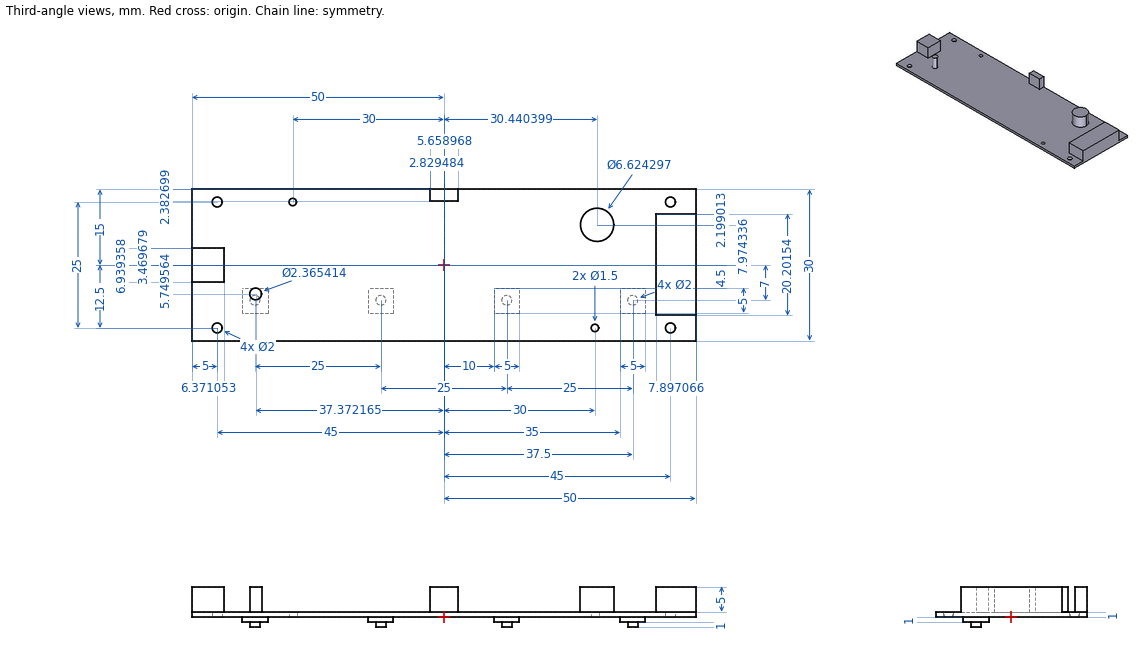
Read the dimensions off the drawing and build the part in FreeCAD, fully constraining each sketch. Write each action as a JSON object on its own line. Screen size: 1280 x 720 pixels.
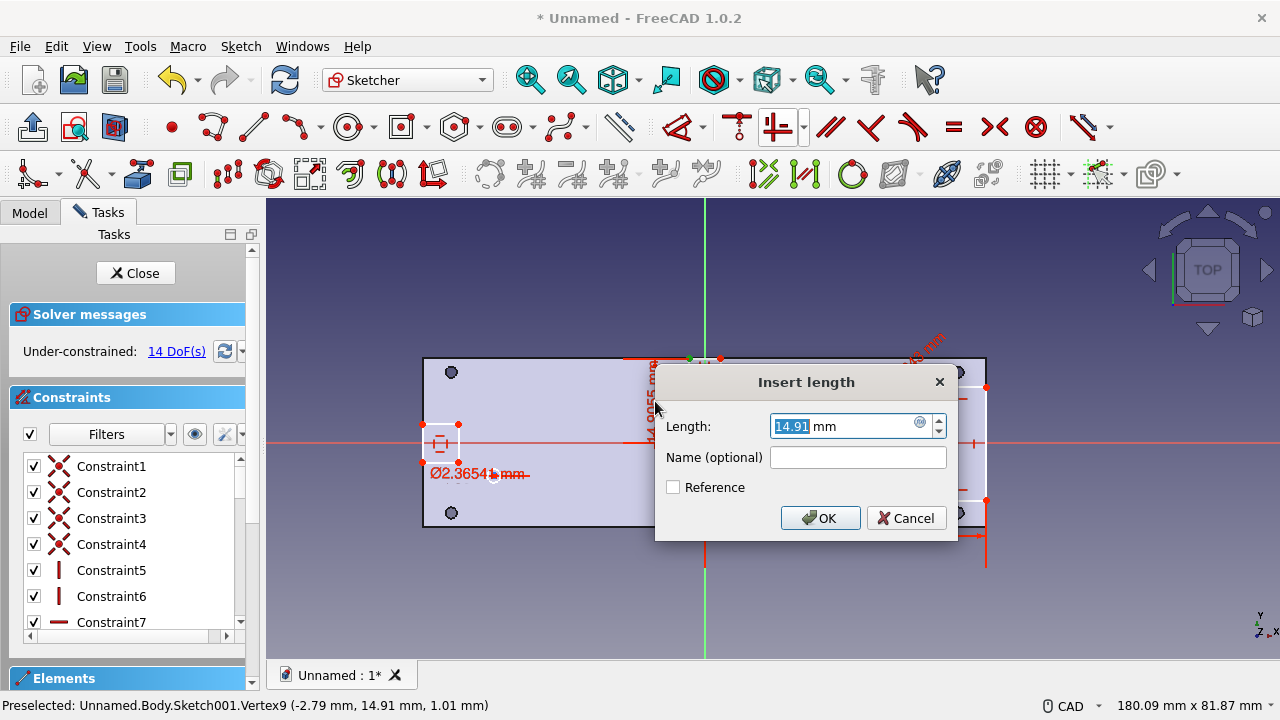
{"action": "type", "text": "15"}
{"action": "key", "text": "Return"}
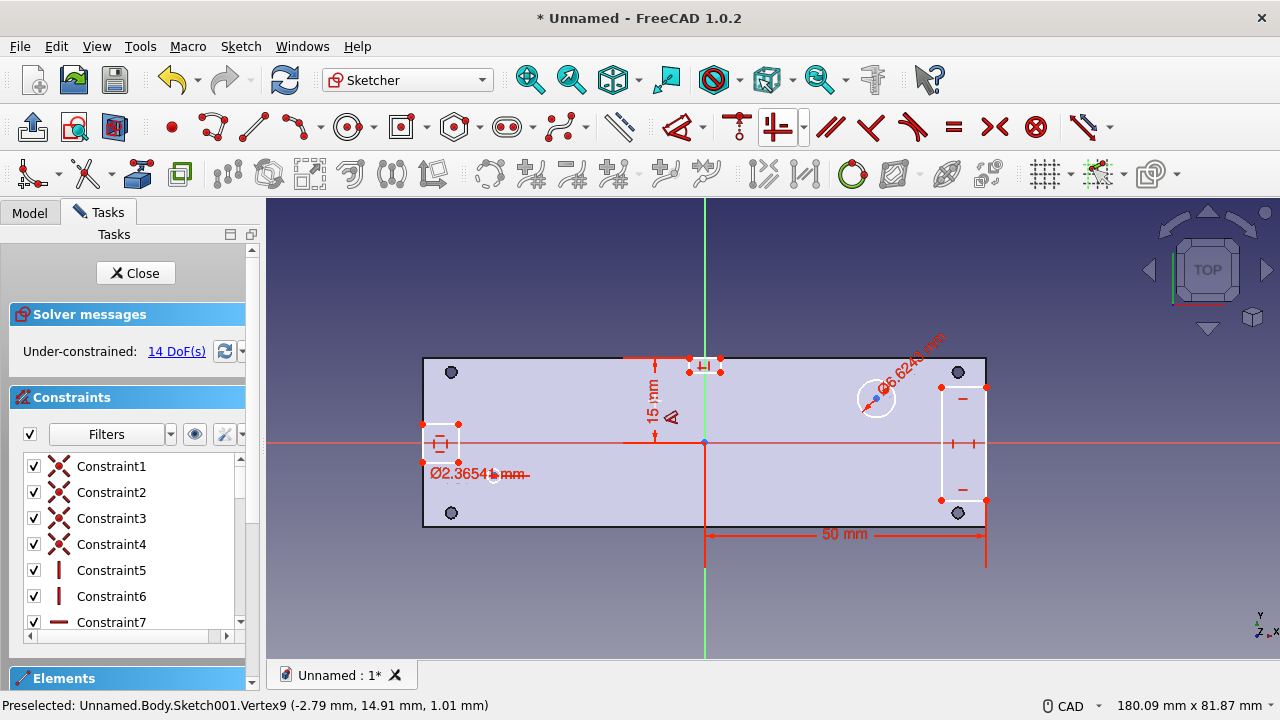
{"action": "left_click", "coordinate": [423, 424]}
{"action": "left_click", "coordinate": [564, 477]}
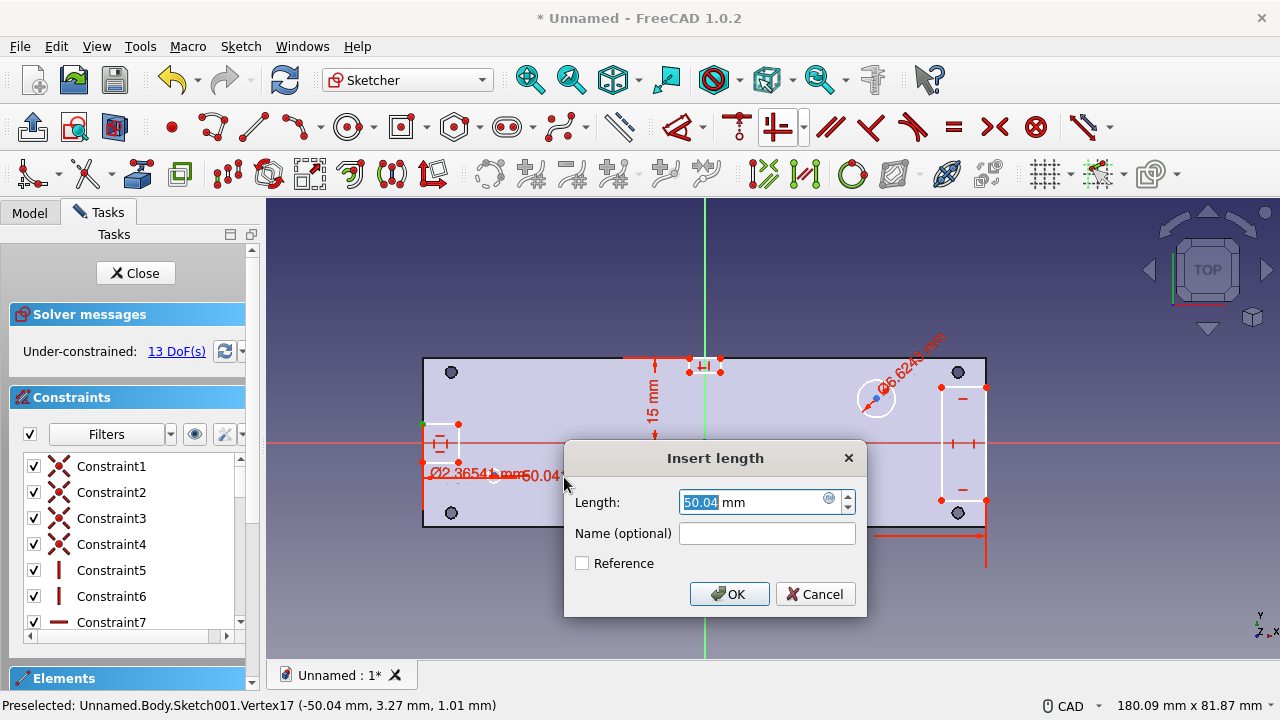
{"action": "type", "text": "50"}
{"action": "key", "text": "Return"}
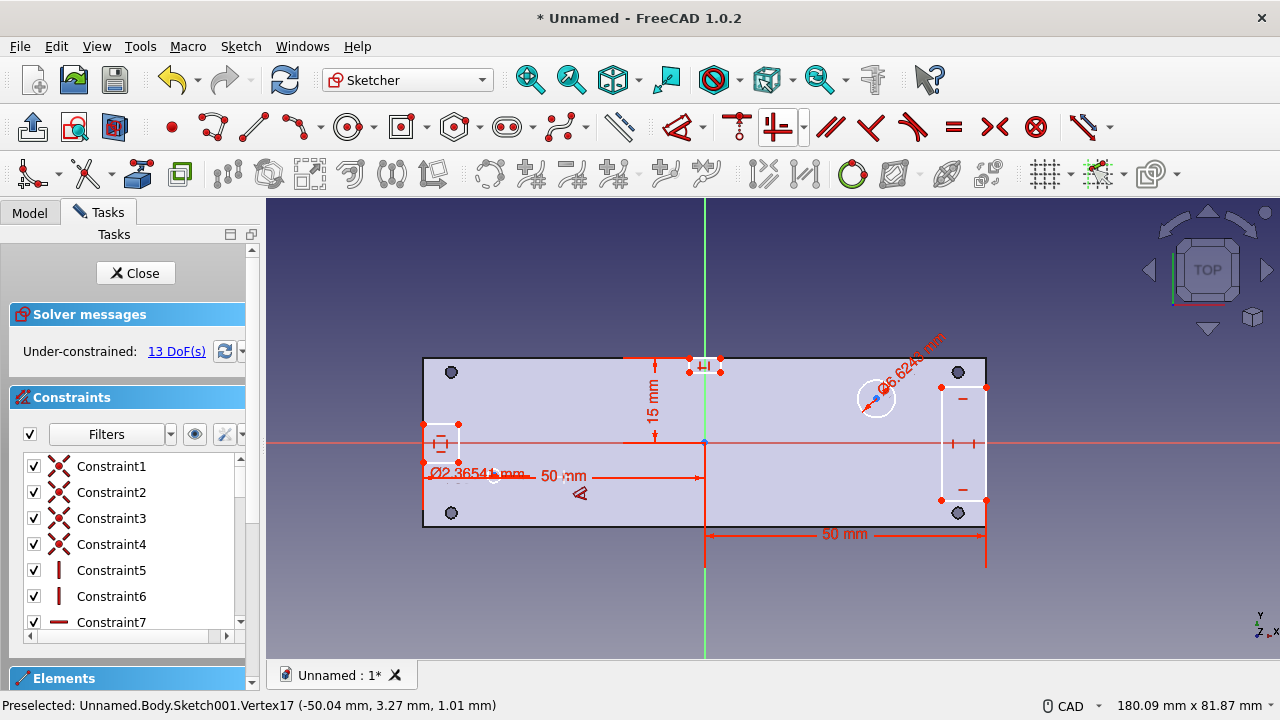
{"action": "left_click", "coordinate": [942, 421]}
{"action": "left_click", "coordinate": [908, 418]}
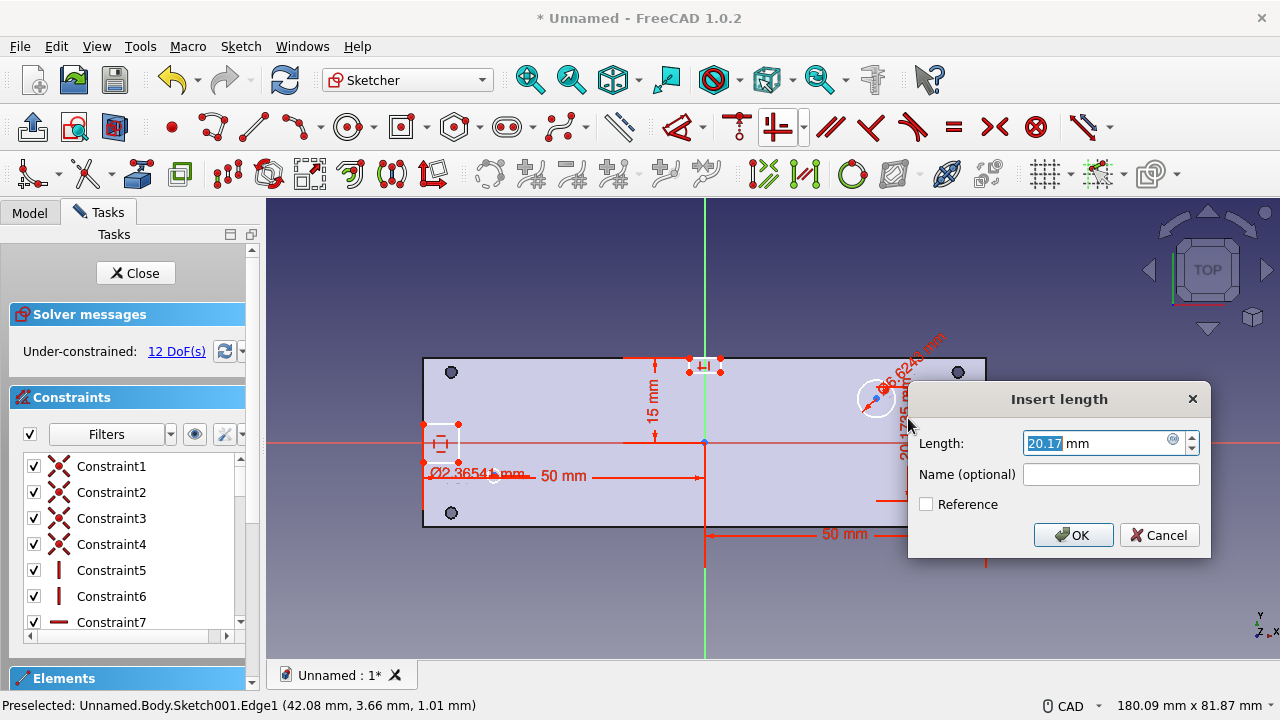
{"action": "type", "text": "20.20154"}
{"action": "key", "text": "Return"}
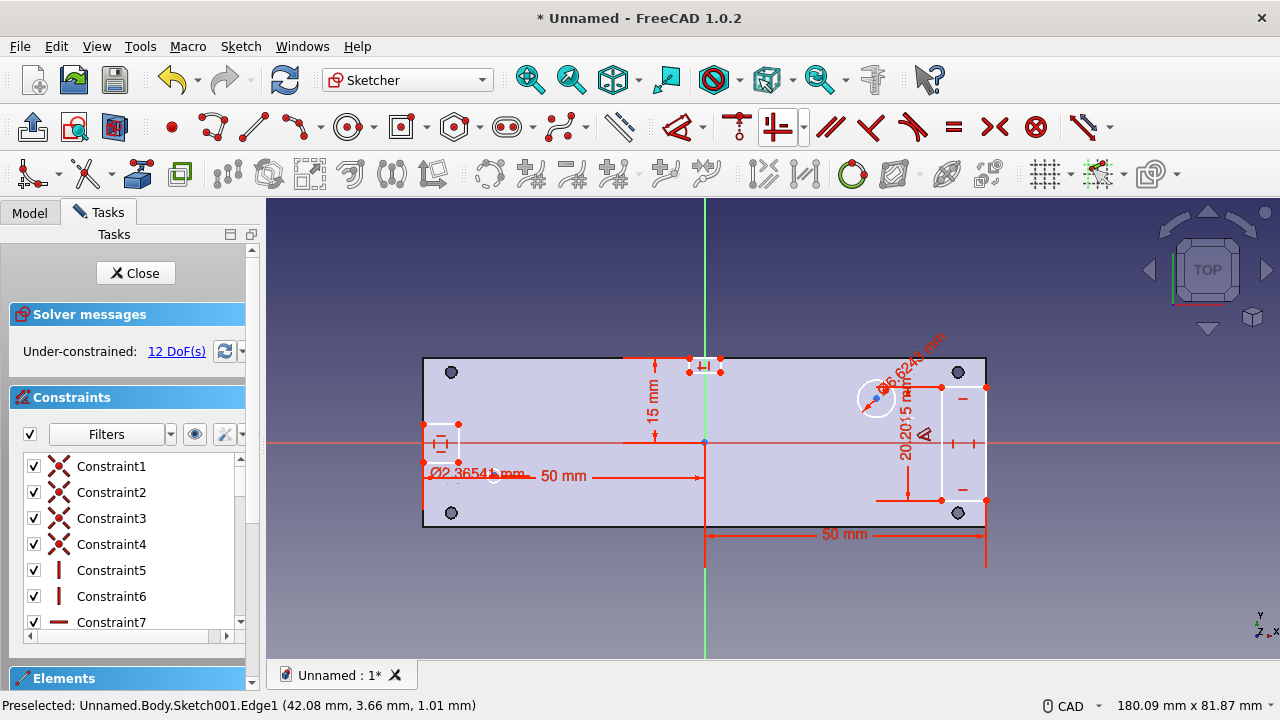
{"action": "left_click", "coordinate": [955, 501]}
{"action": "left_click", "coordinate": [964, 535]}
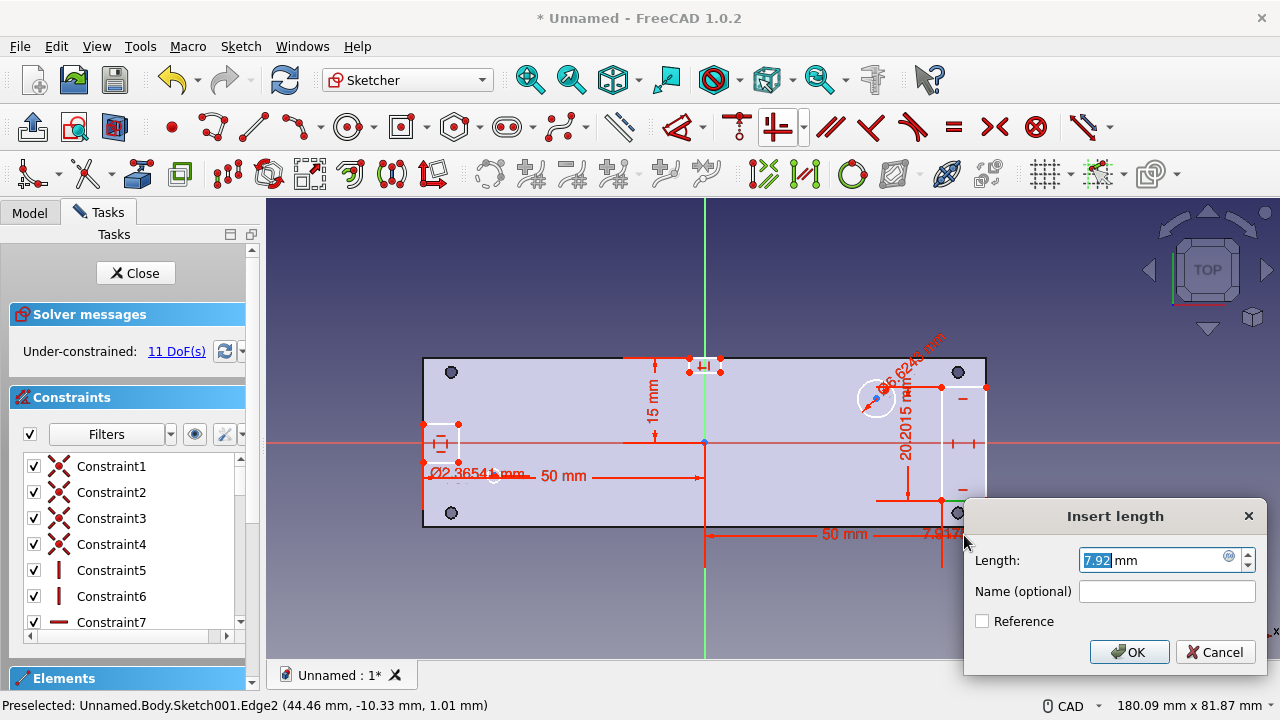
{"action": "type", "text": "7.897066"}
{"action": "key", "text": "Return"}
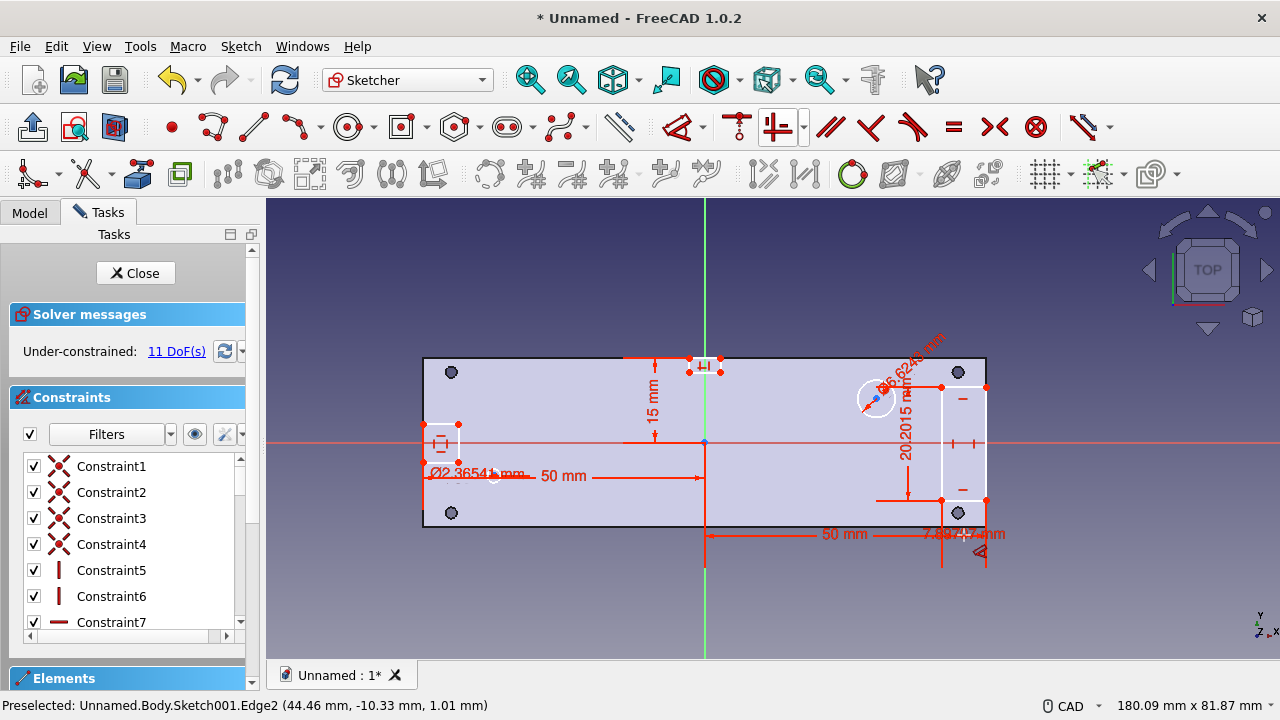
{"action": "scroll", "coordinate": [689, 365], "scroll_direction": "up", "scroll_amount": 6}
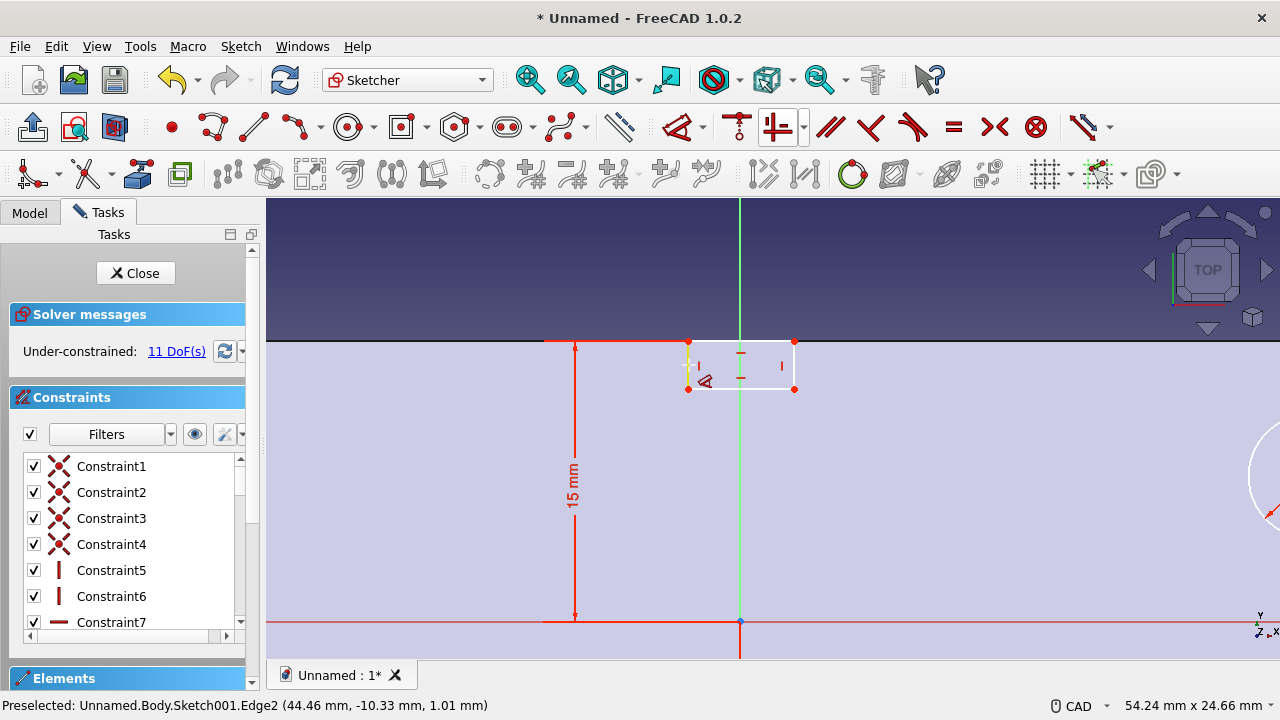
{"action": "left_click", "coordinate": [688, 365]}
{"action": "left_click", "coordinate": [654, 365]}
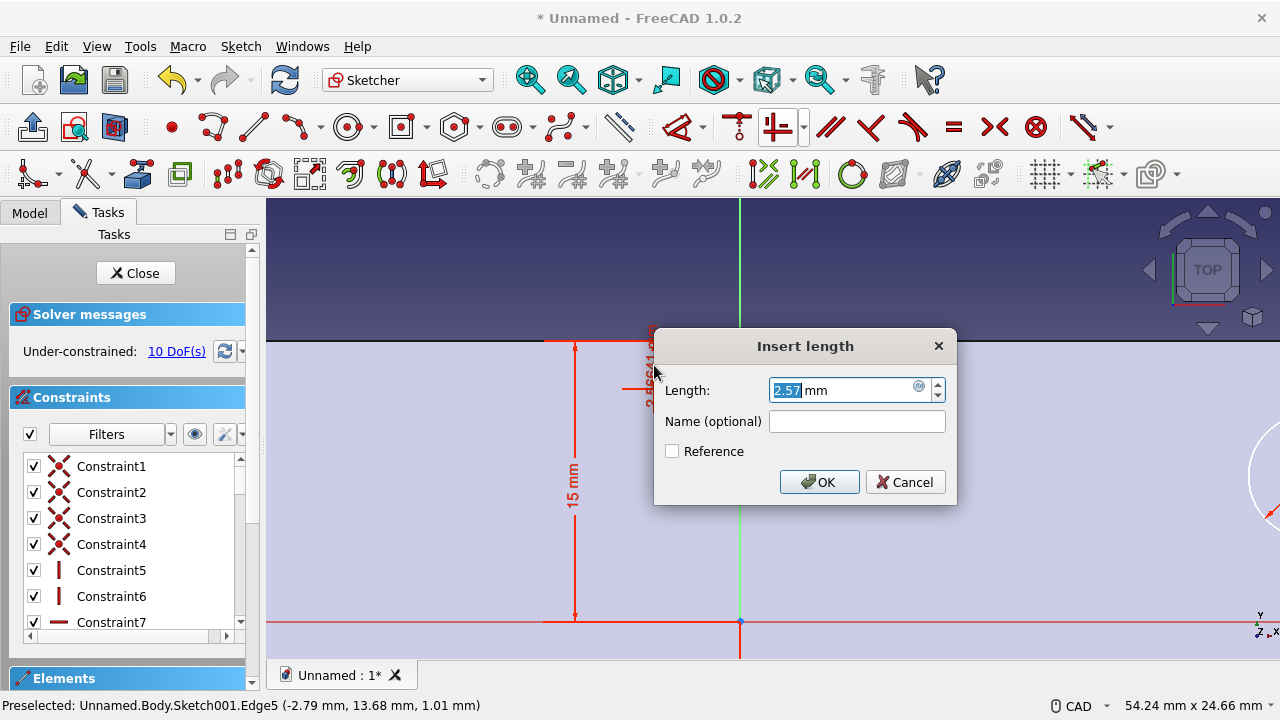
{"action": "type", "text": "2.382699"}
{"action": "key", "text": "Return"}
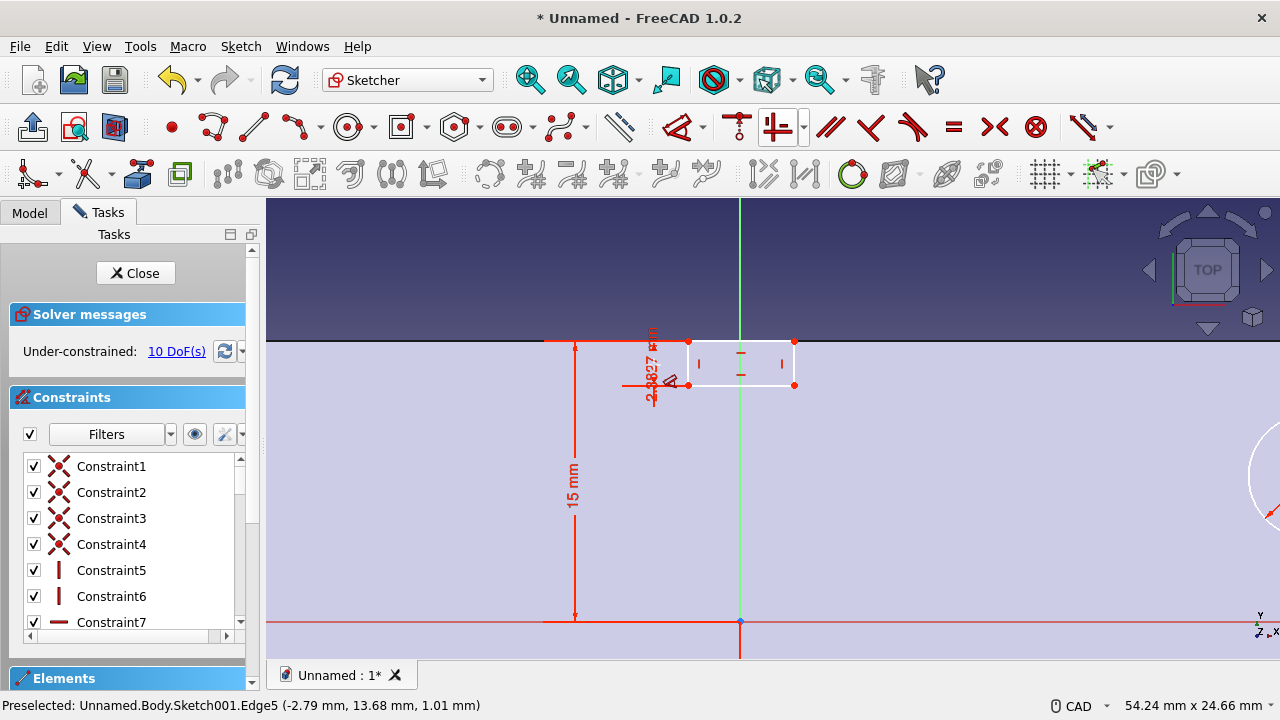
{"action": "left_click", "coordinate": [720, 386]}
{"action": "left_click", "coordinate": [717, 420]}